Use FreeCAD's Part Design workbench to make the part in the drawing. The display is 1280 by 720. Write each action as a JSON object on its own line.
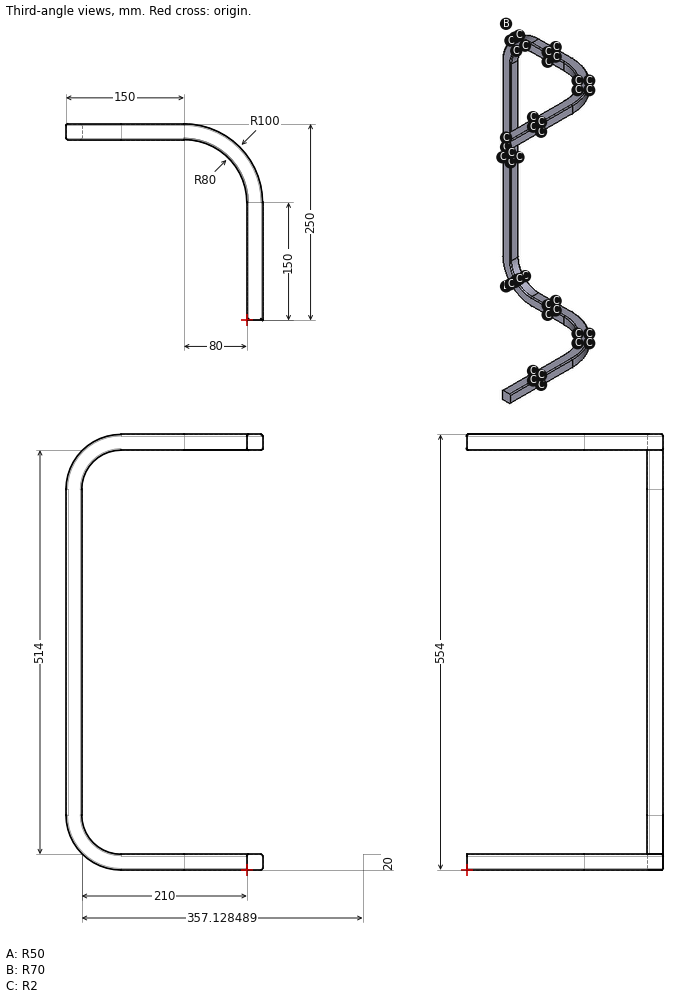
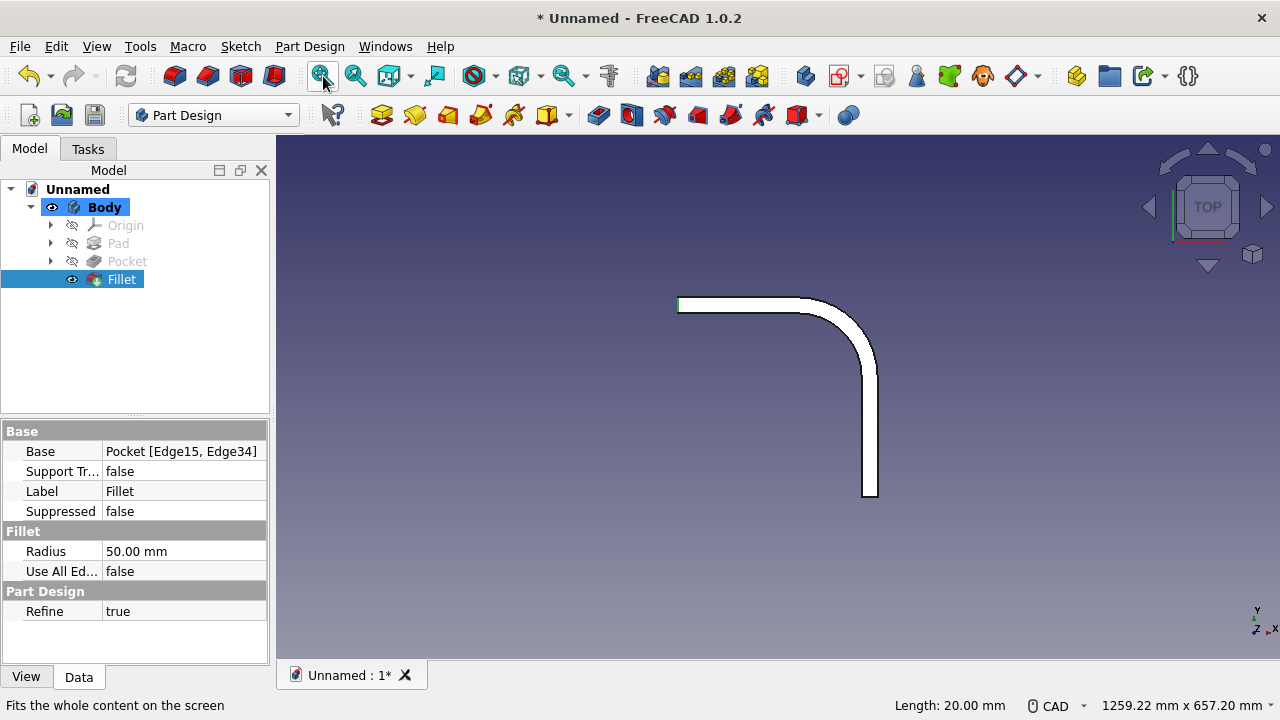
{"action": "key", "text": "1"}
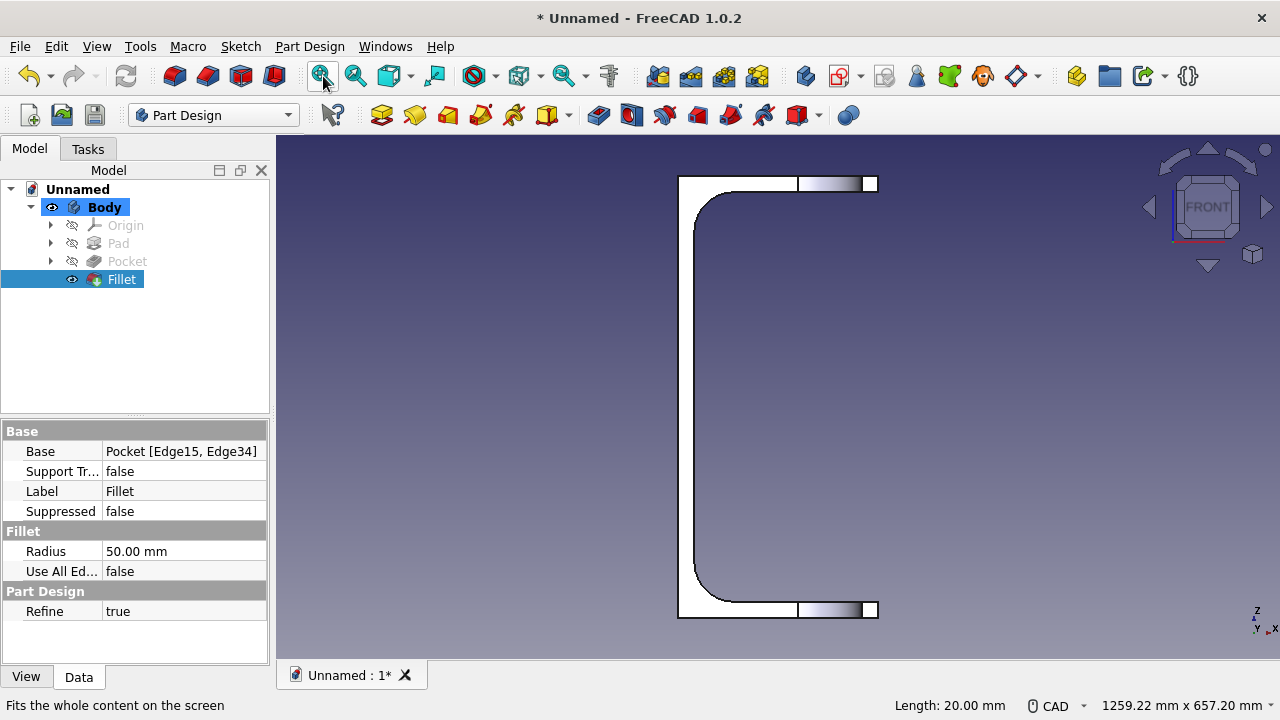
{"action": "scroll", "coordinate": [678, 617], "scroll_direction": "up", "scroll_amount": 5}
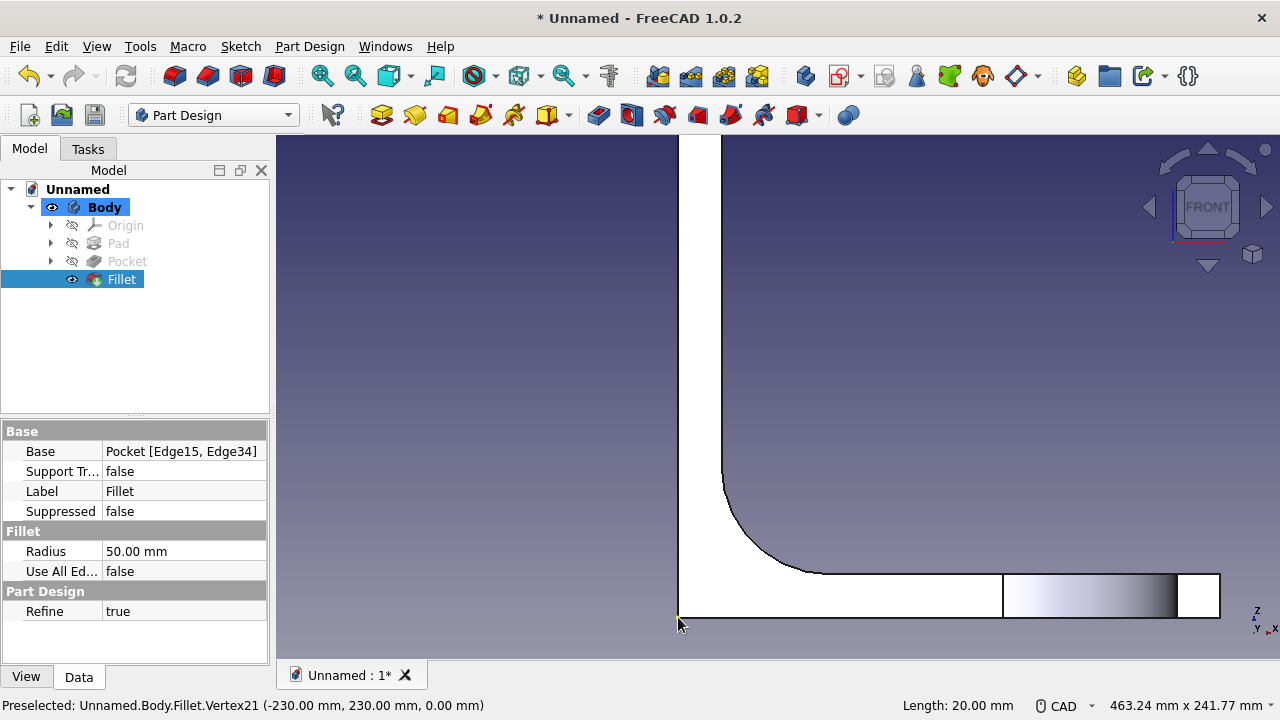
{"action": "left_click", "coordinate": [323, 76]}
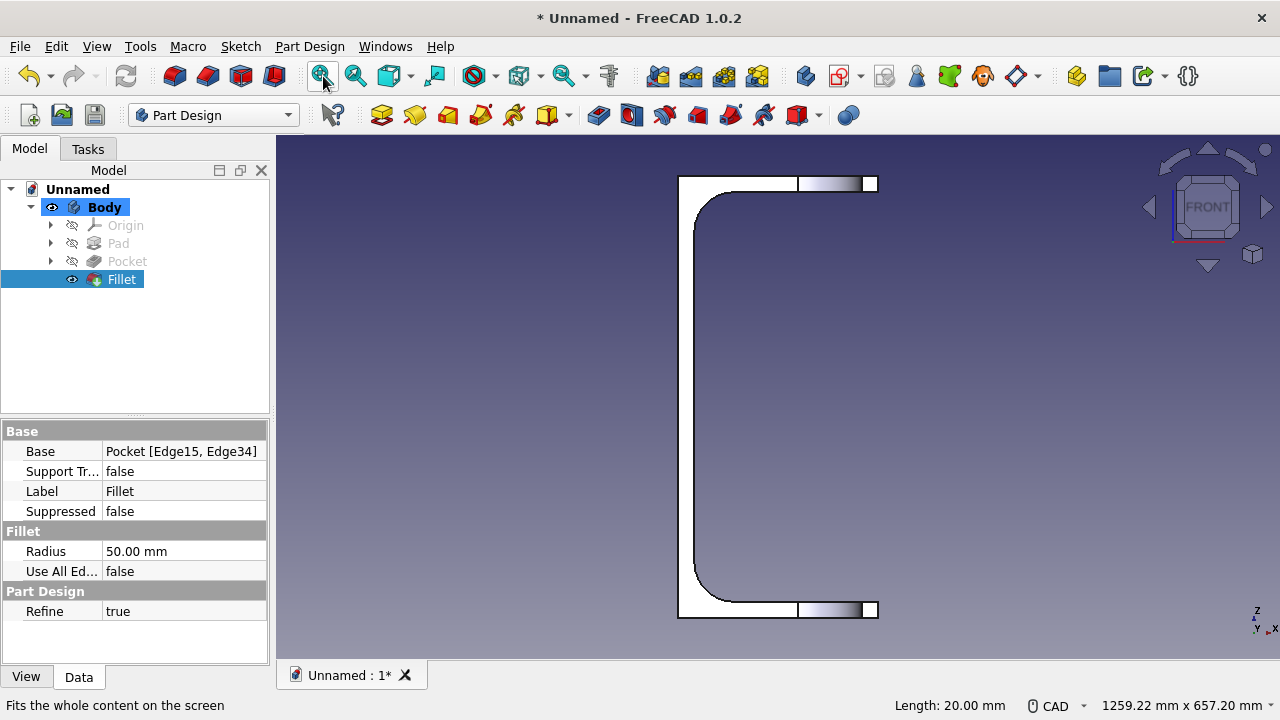
{"action": "key", "text": "3"}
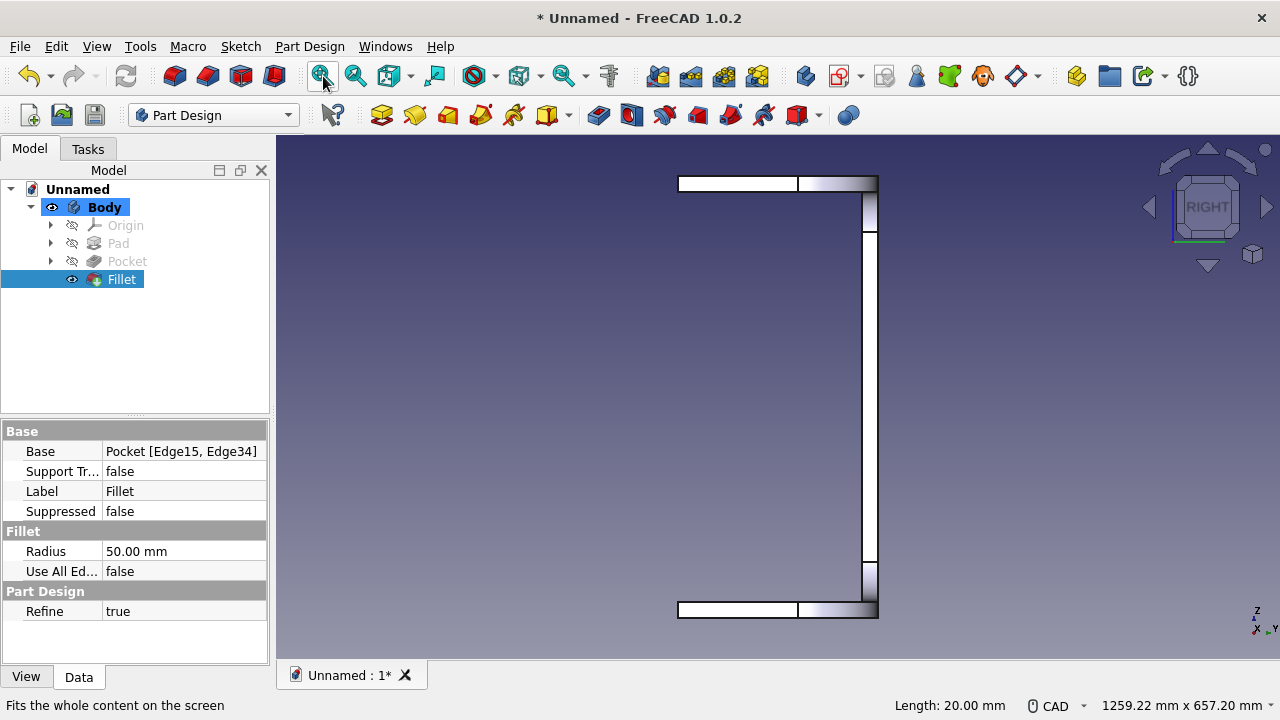
{"action": "scroll", "coordinate": [870, 617], "scroll_direction": "up", "scroll_amount": 5}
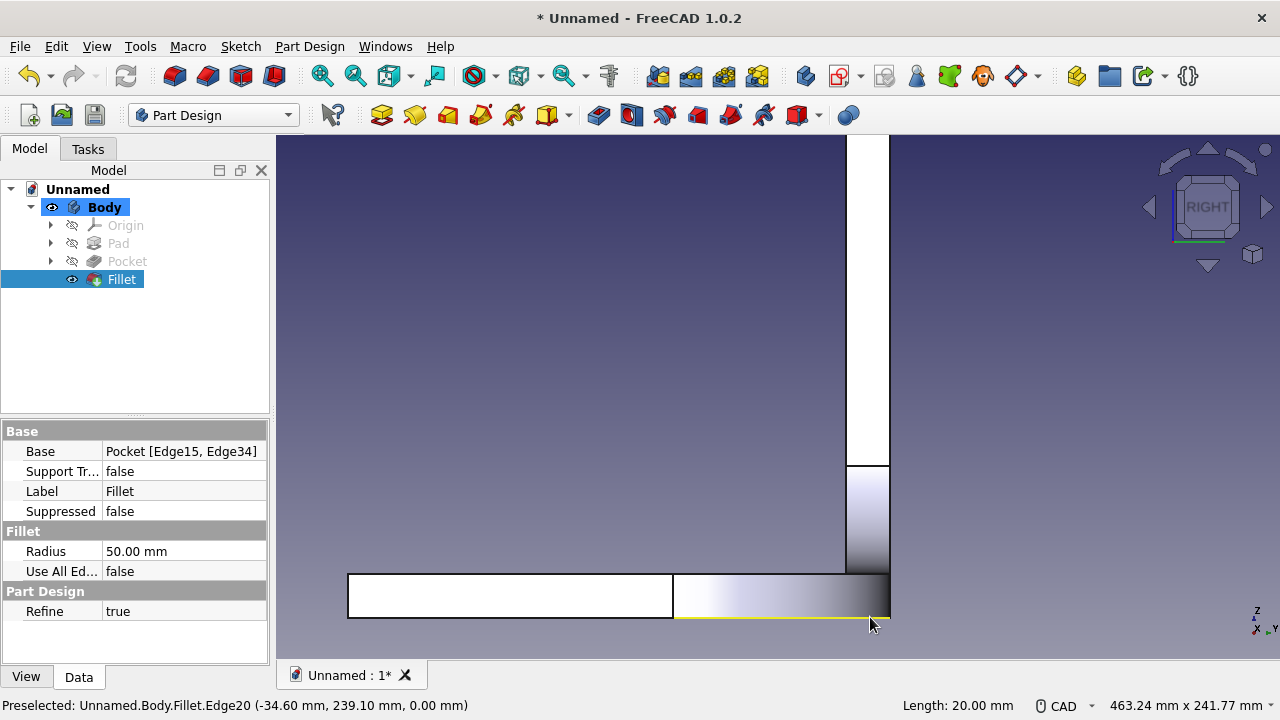
{"action": "left_click", "coordinate": [323, 76]}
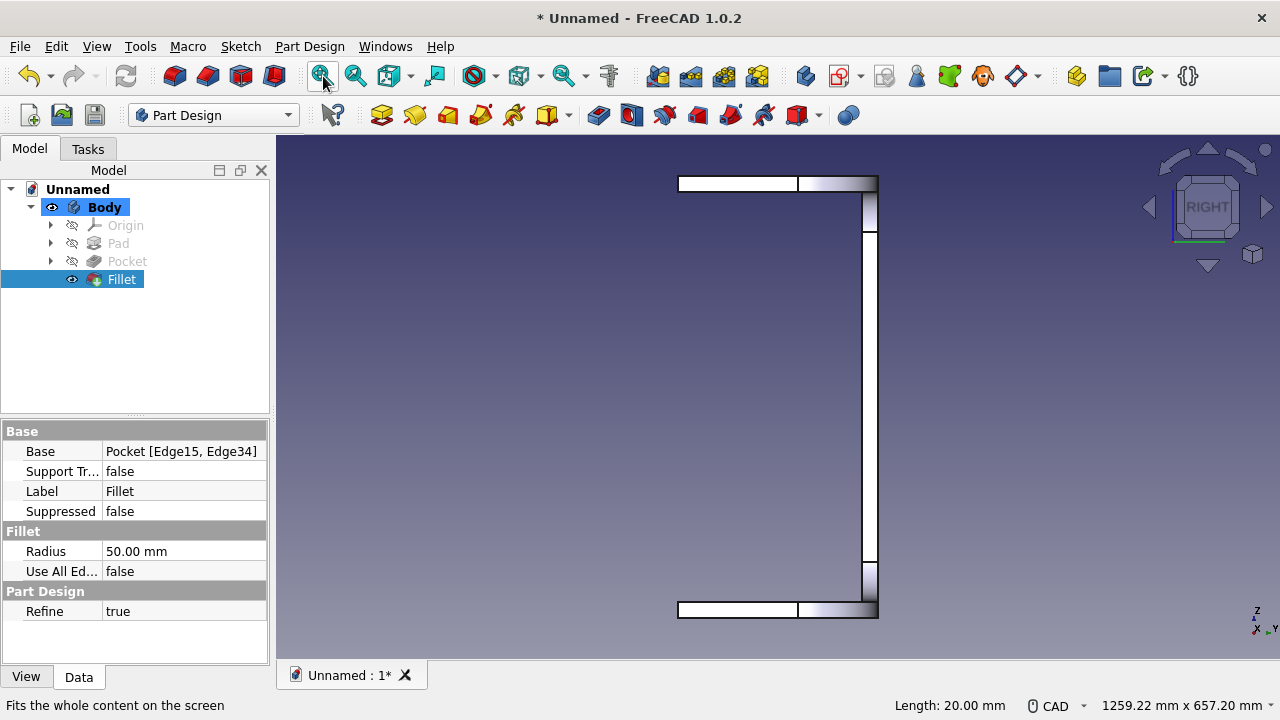
{"action": "key", "text": "5"}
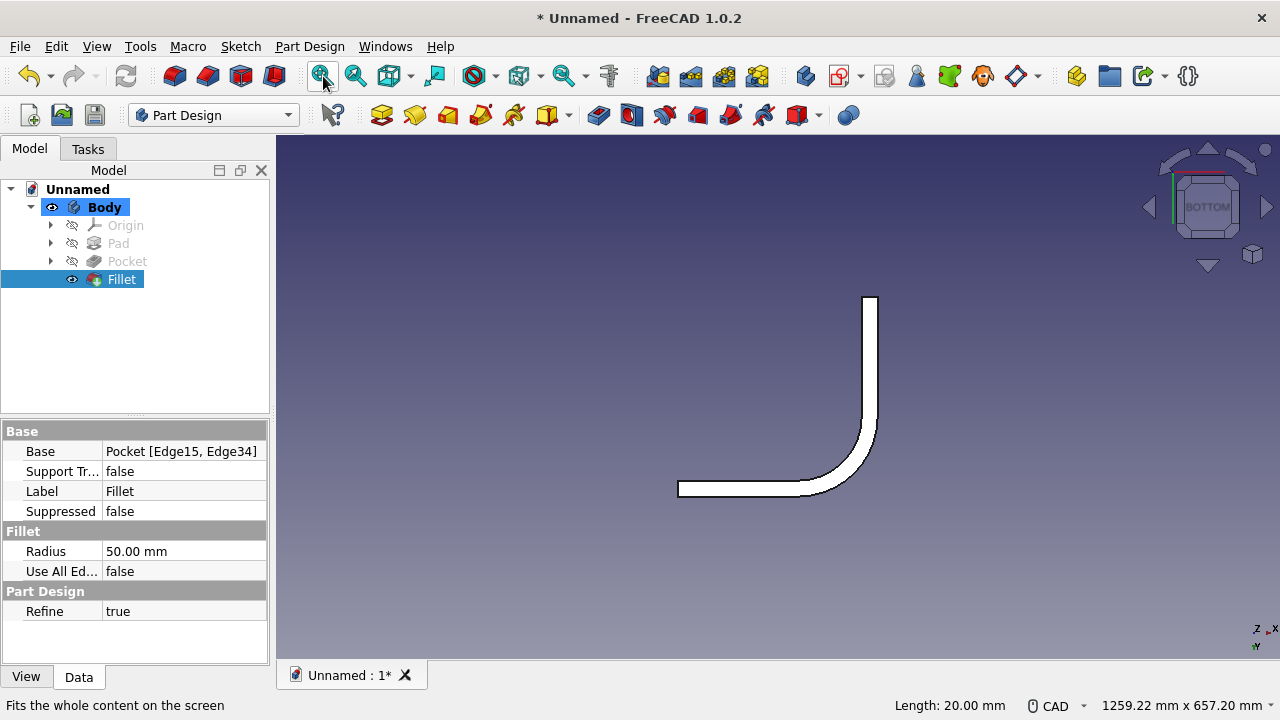
{"action": "left_click", "coordinate": [323, 76]}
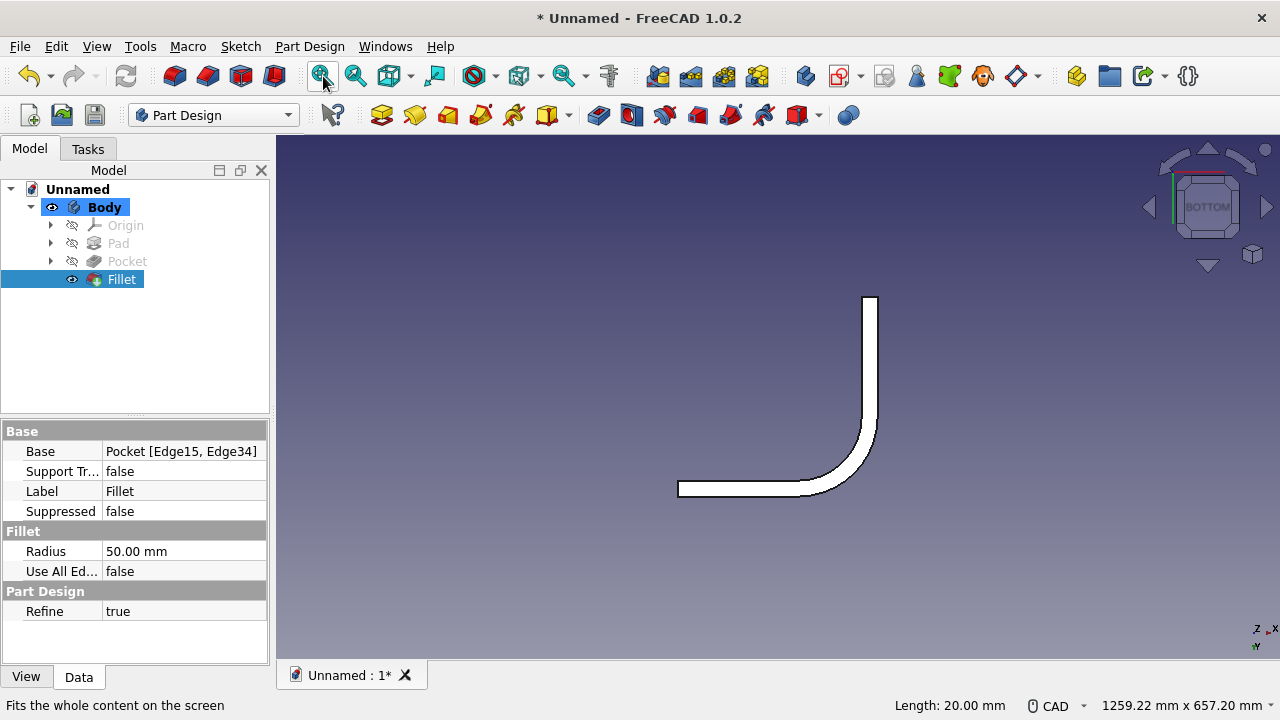
{"action": "left_click", "coordinate": [678, 488], "text": "ctrl"}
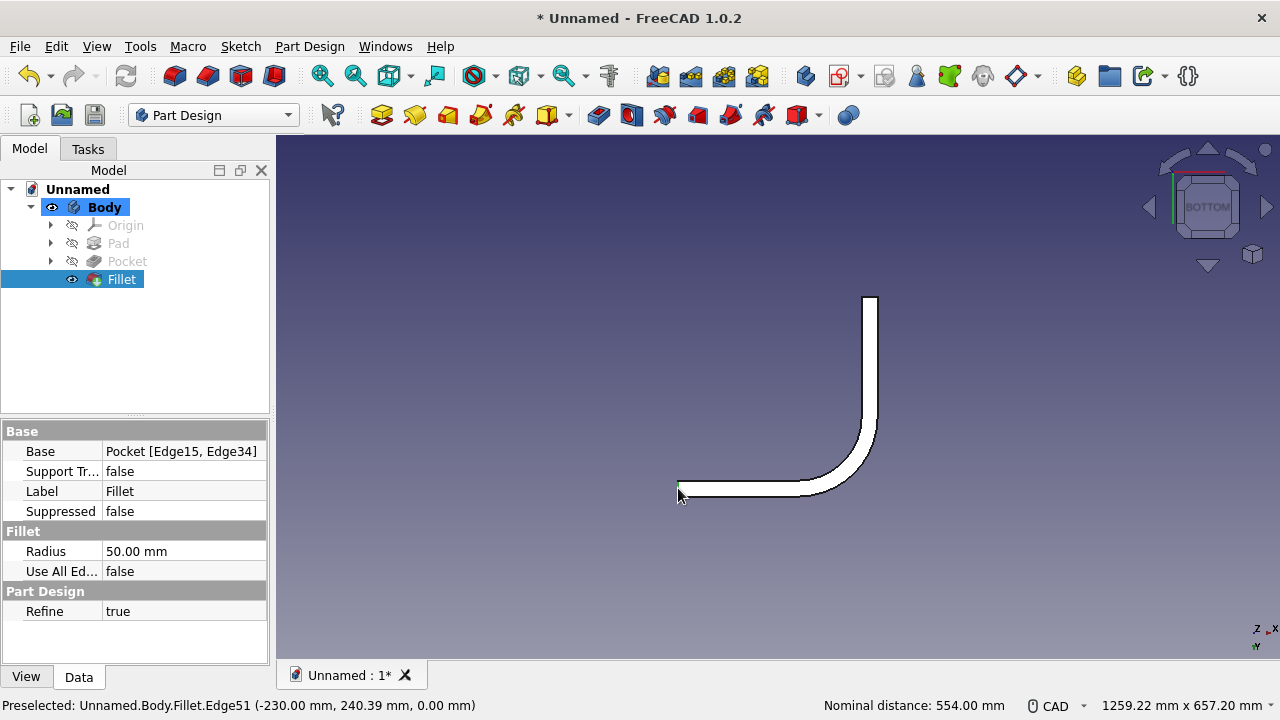
{"action": "left_click", "coordinate": [175, 76]}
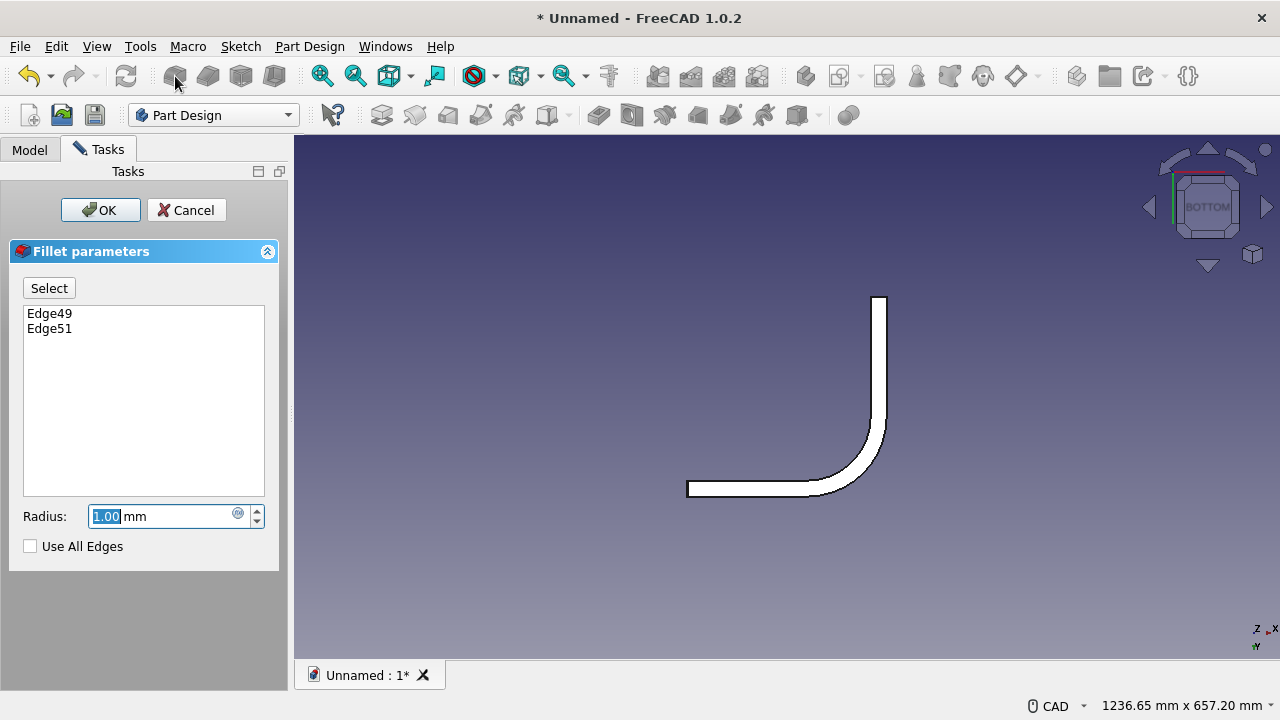
{"action": "type", "text": "70"}
{"action": "key", "text": "Tab"}